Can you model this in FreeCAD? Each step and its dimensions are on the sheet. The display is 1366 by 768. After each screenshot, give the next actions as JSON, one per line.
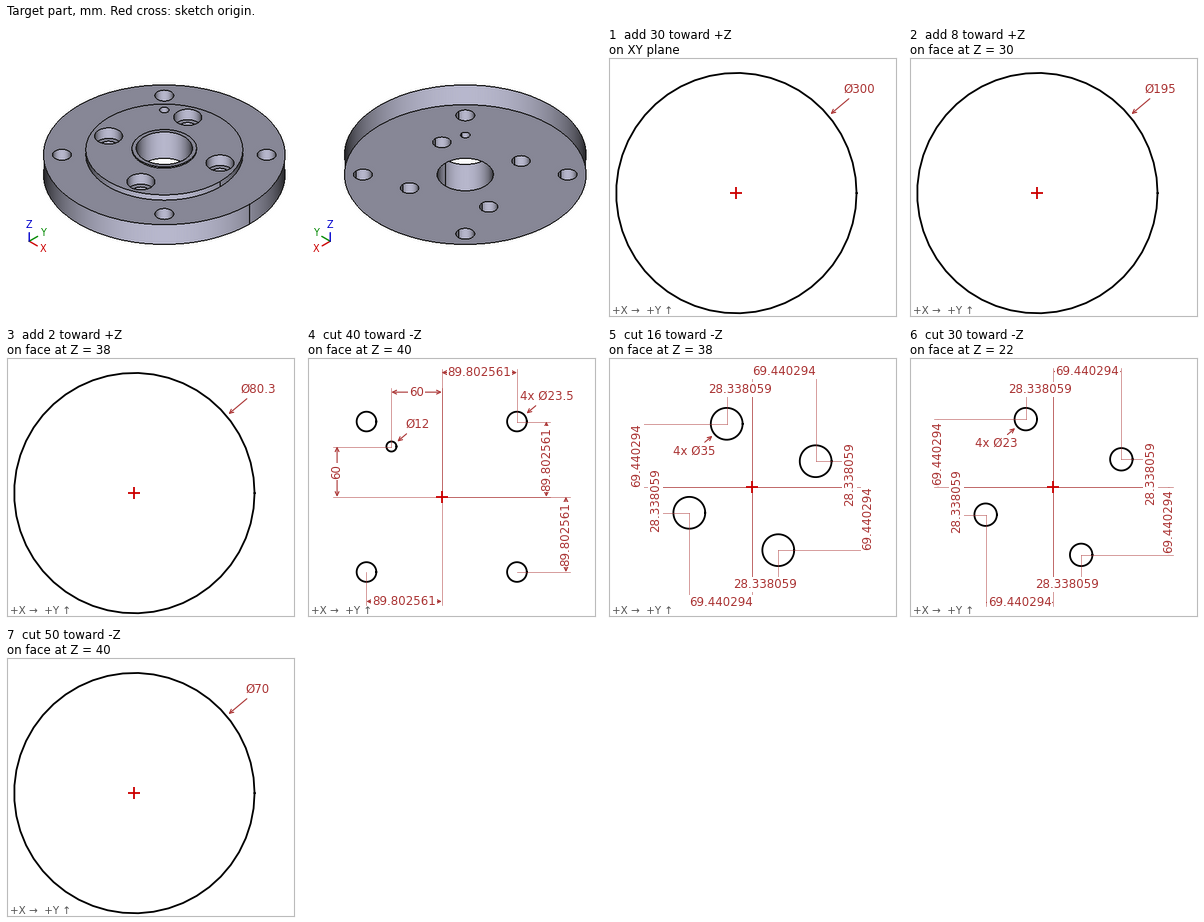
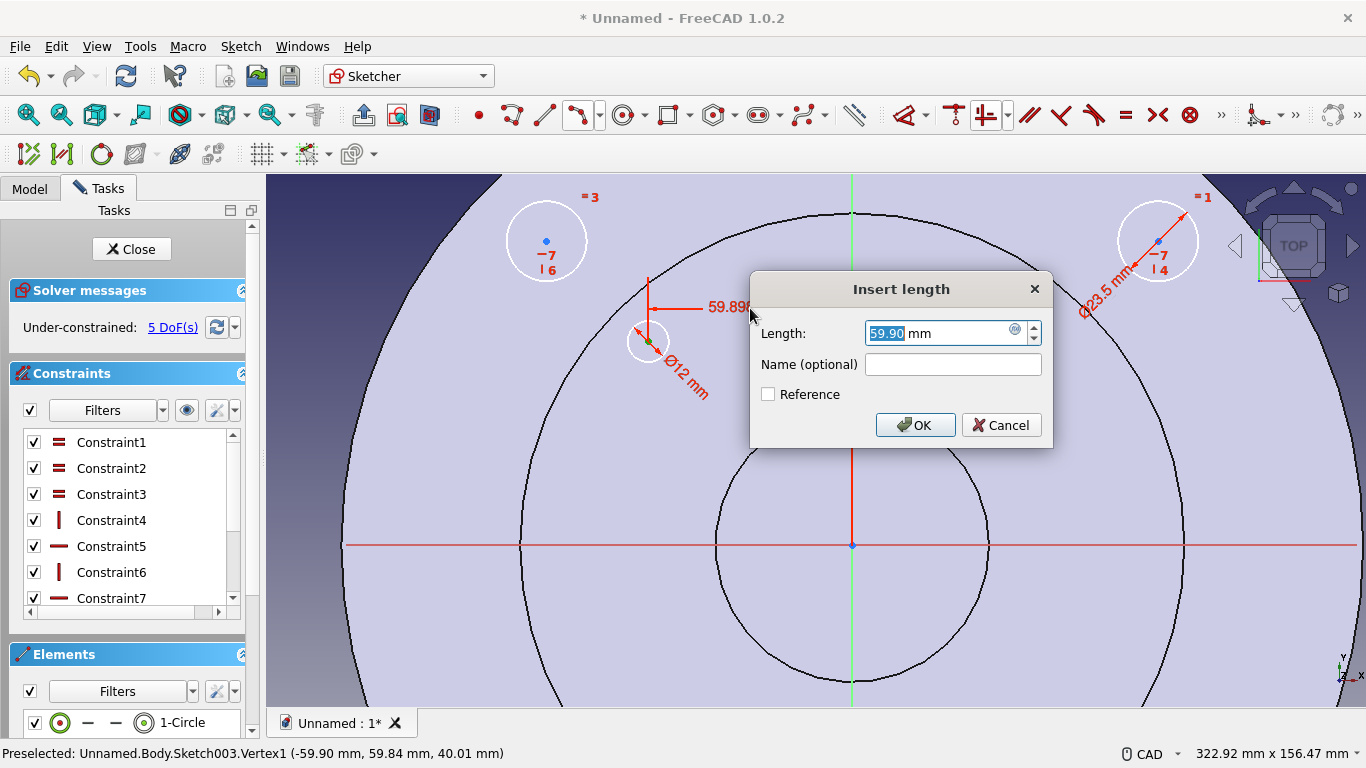
{"action": "type", "text": "60"}
{"action": "key", "text": "Return"}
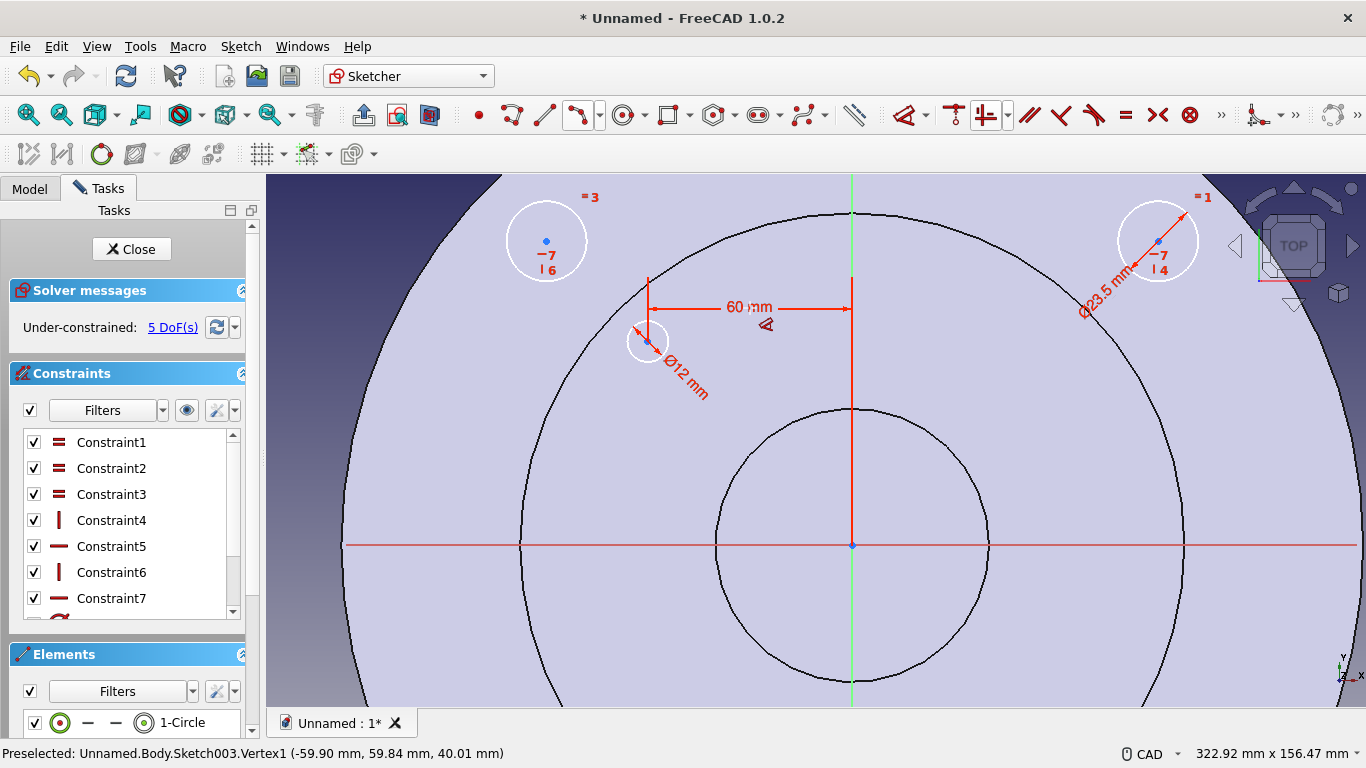
{"action": "left_click", "coordinate": [648, 342]}
{"action": "left_click", "coordinate": [614, 443]}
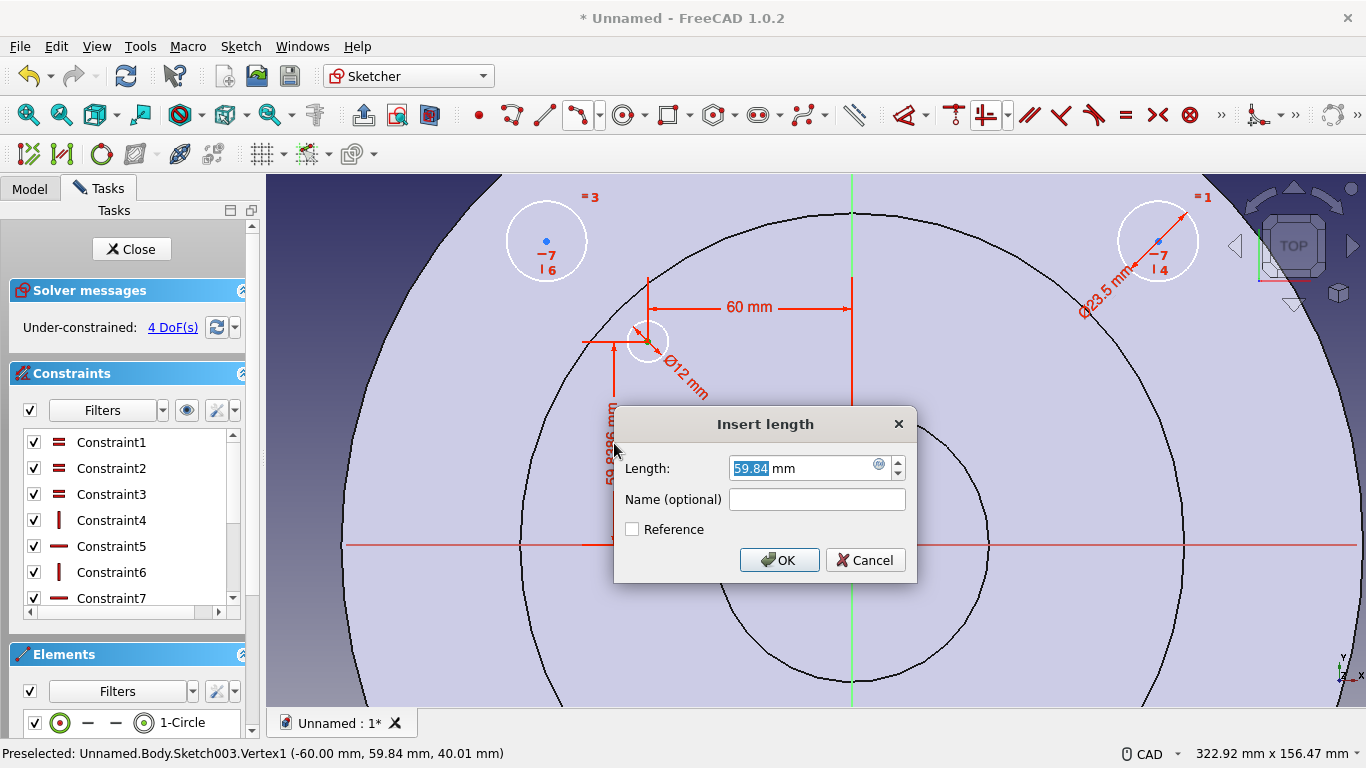
{"action": "type", "text": "60"}
{"action": "key", "text": "Return"}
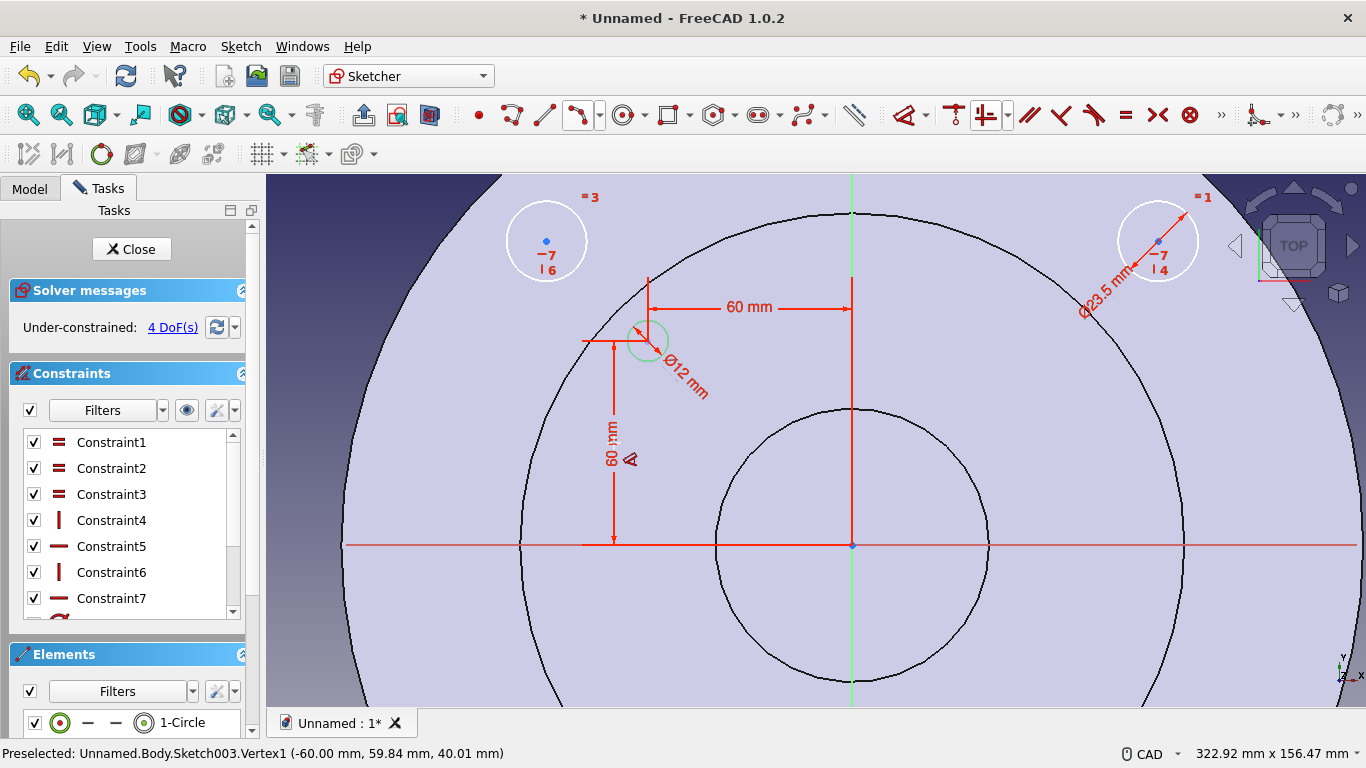
{"action": "left_click", "coordinate": [1158, 241]}
{"action": "left_click", "coordinate": [1005, 207]}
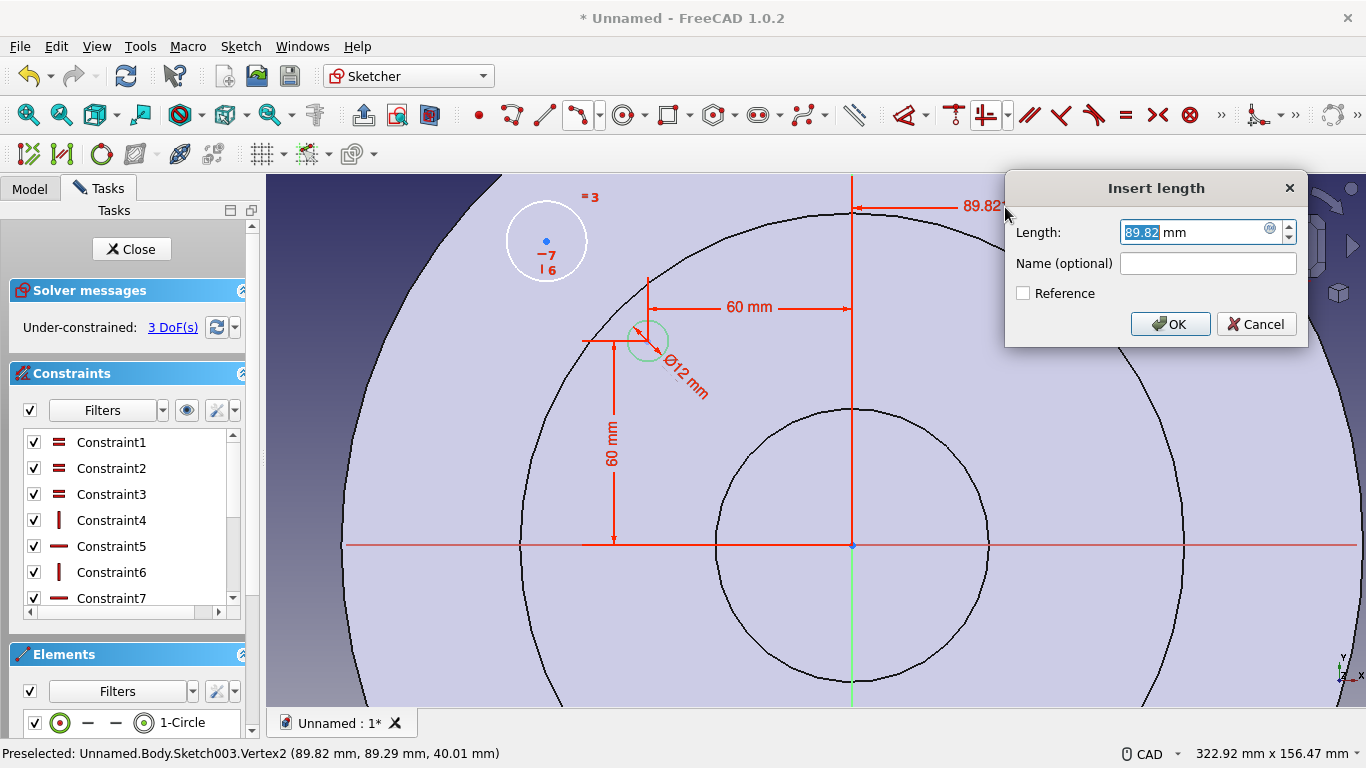
{"action": "type", "text": "89.802561"}
{"action": "key", "text": "Return"}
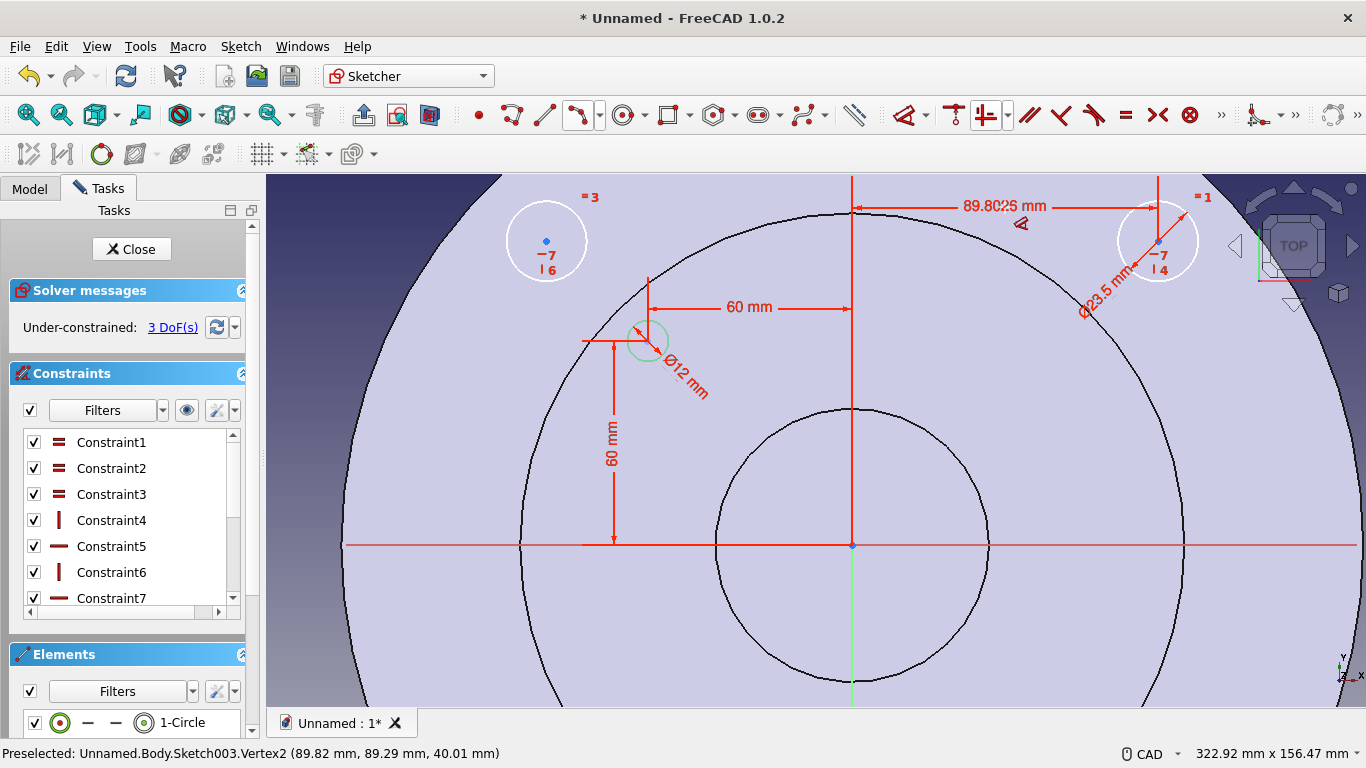
{"action": "left_click", "coordinate": [1158, 241]}
{"action": "left_click", "coordinate": [1192, 393]}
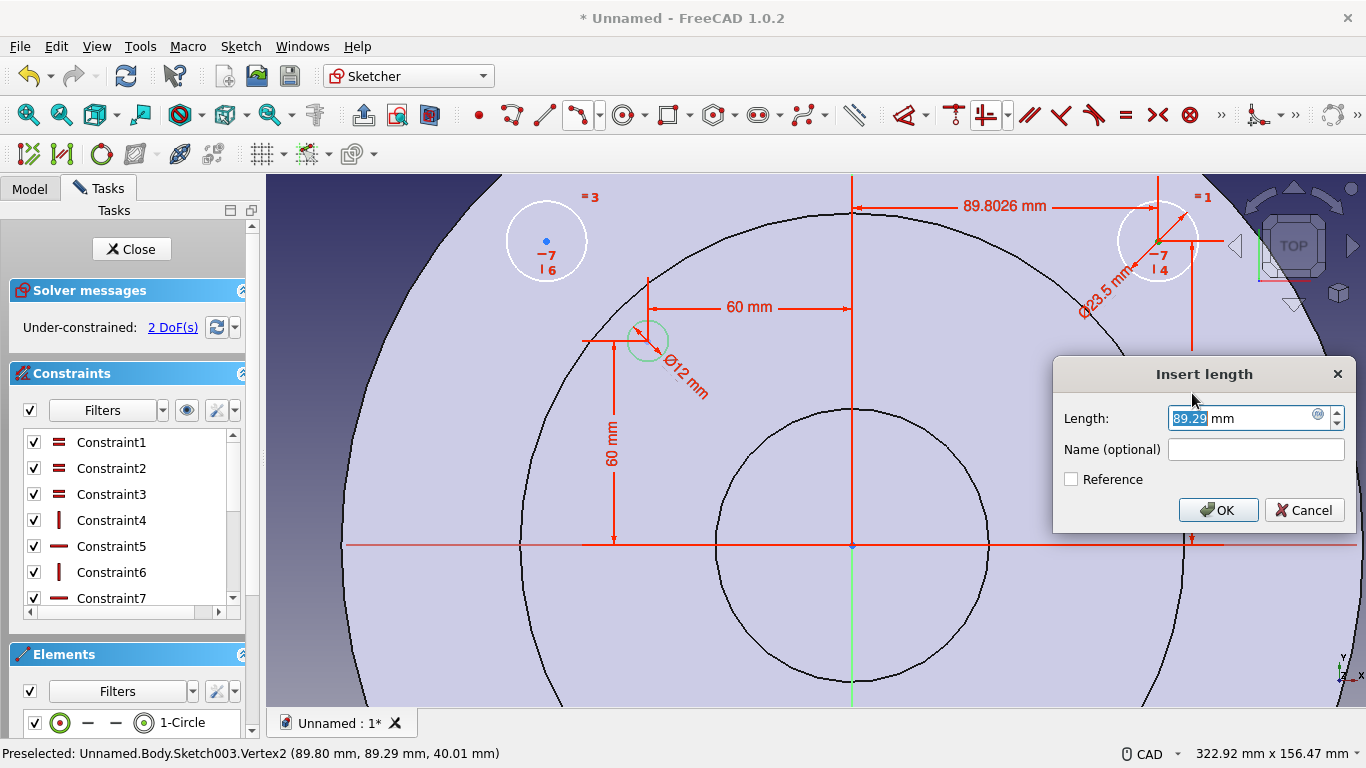
{"action": "type", "text": "89.802561"}
{"action": "key", "text": "Return"}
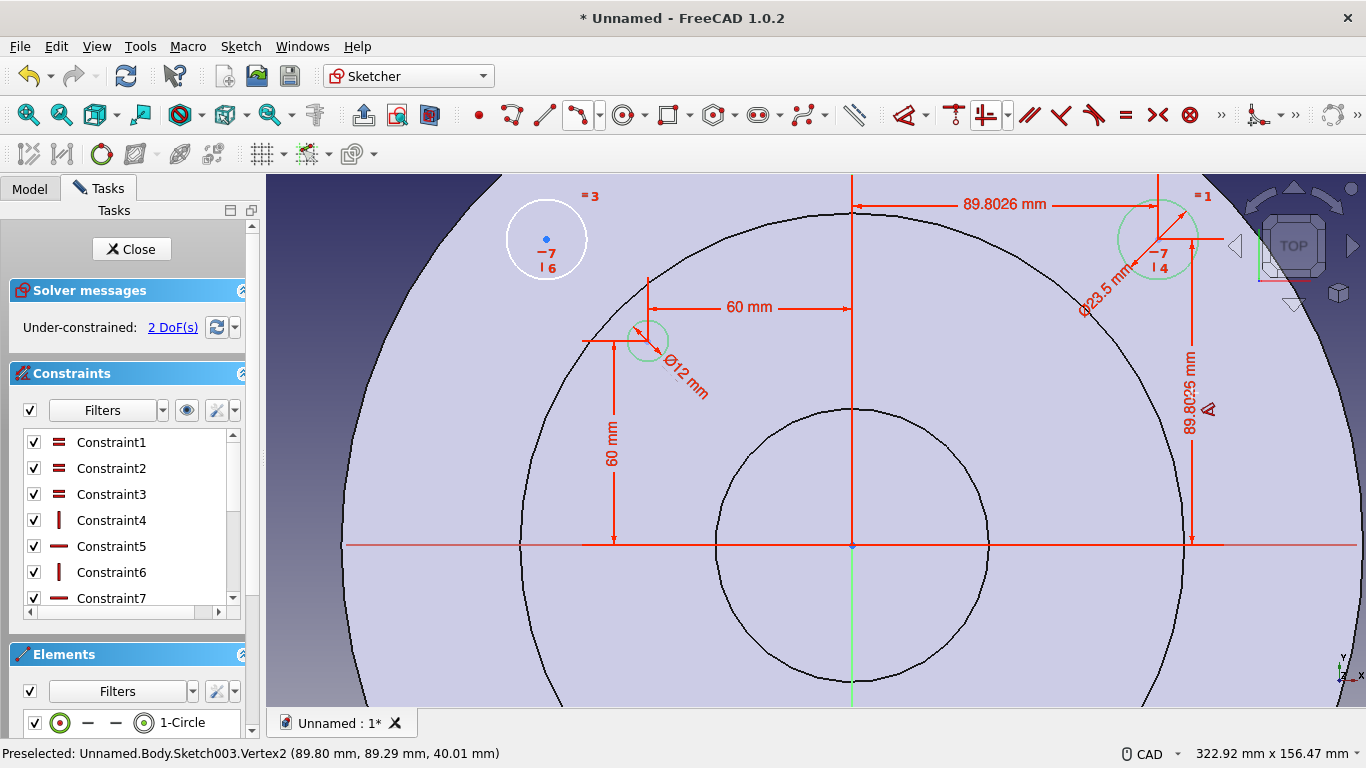
{"action": "scroll", "coordinate": [662, 355], "scroll_direction": "down", "scroll_amount": 4}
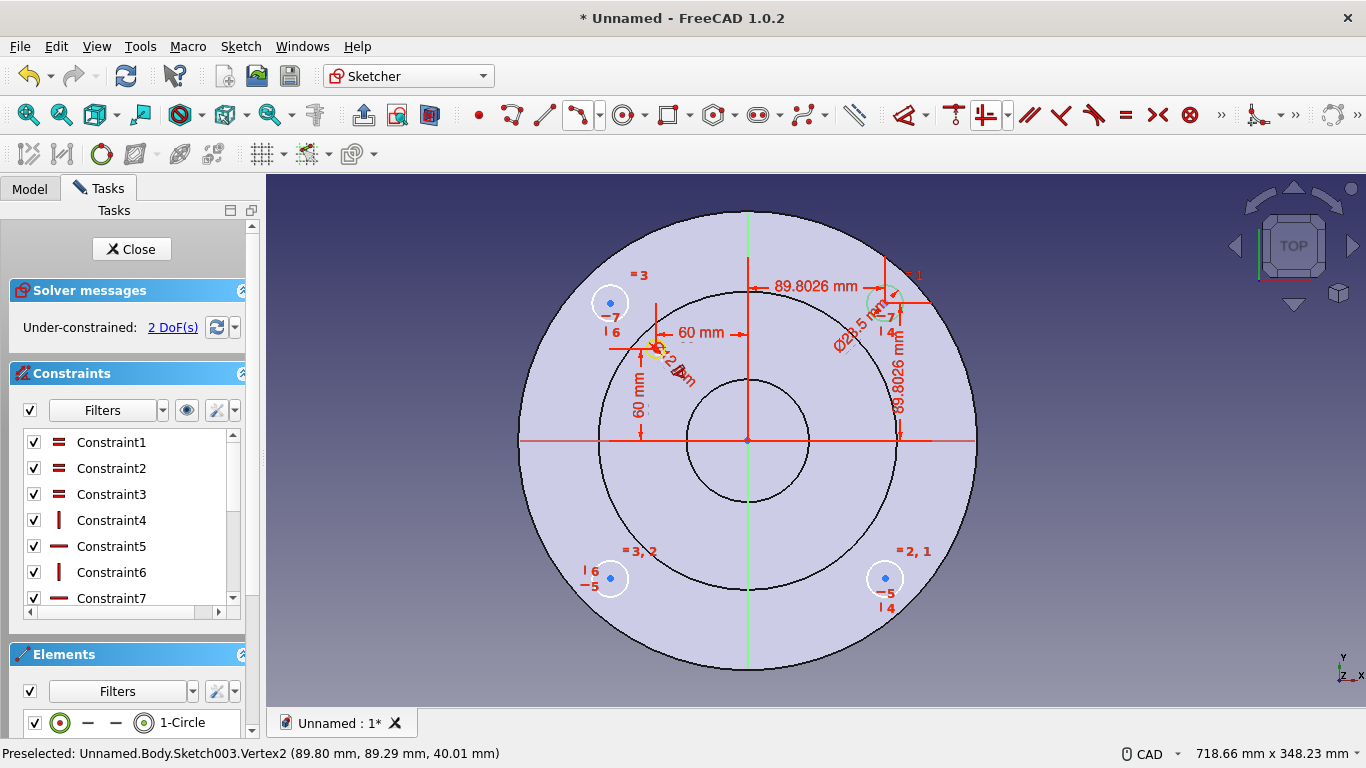
{"action": "left_click", "coordinate": [885, 579]}
{"action": "left_click", "coordinate": [919, 510]}